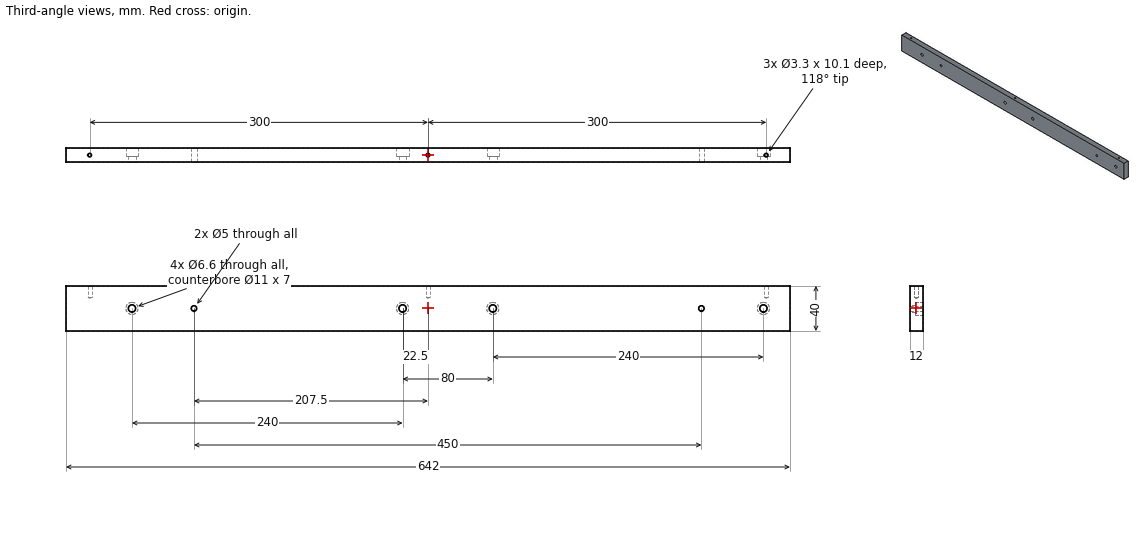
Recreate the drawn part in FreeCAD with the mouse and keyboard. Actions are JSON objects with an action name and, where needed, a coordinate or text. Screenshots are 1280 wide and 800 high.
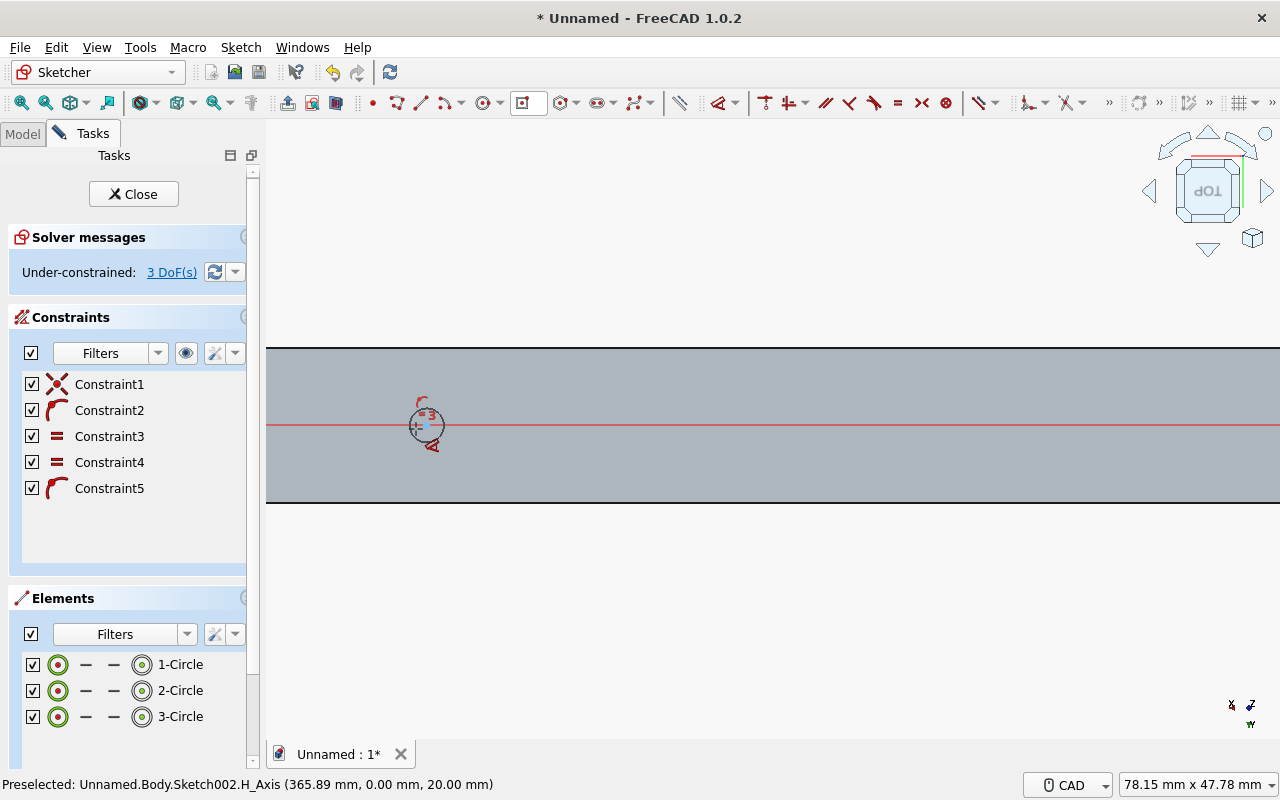
{"action": "left_click", "coordinate": [410, 425]}
{"action": "left_click", "coordinate": [385, 401]}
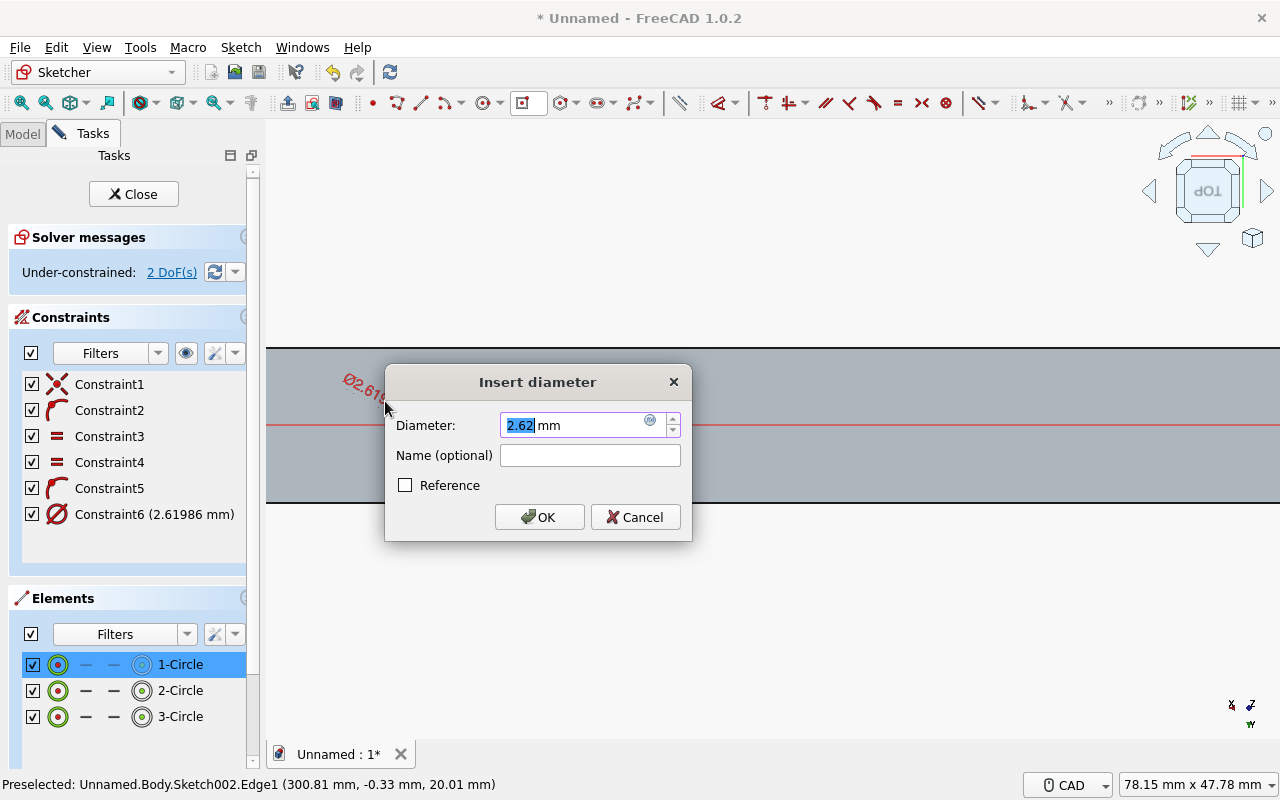
{"action": "type", "text": "3.3"}
{"action": "key", "text": "Return"}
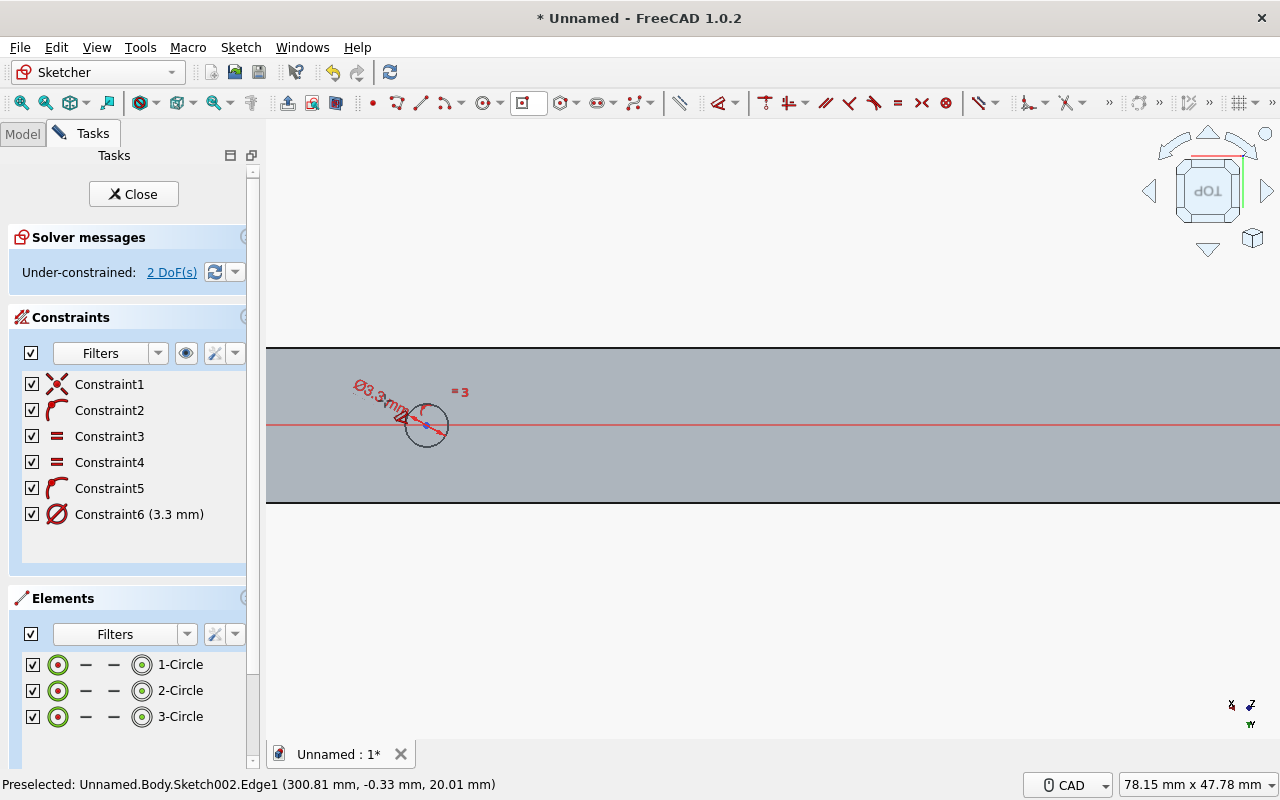
{"action": "scroll", "coordinate": [415, 429], "scroll_direction": "down", "scroll_amount": 13}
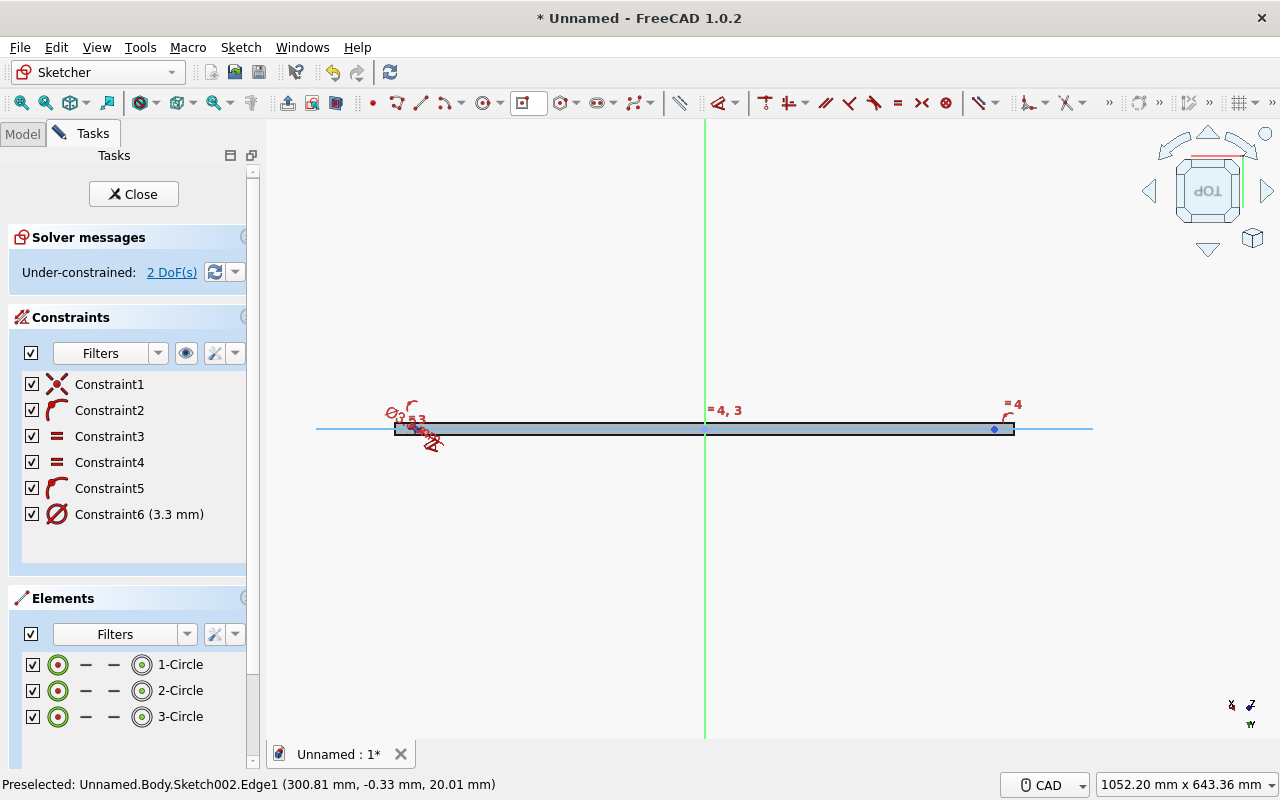
{"action": "left_click", "coordinate": [416, 429]}
{"action": "left_click", "coordinate": [560, 463]}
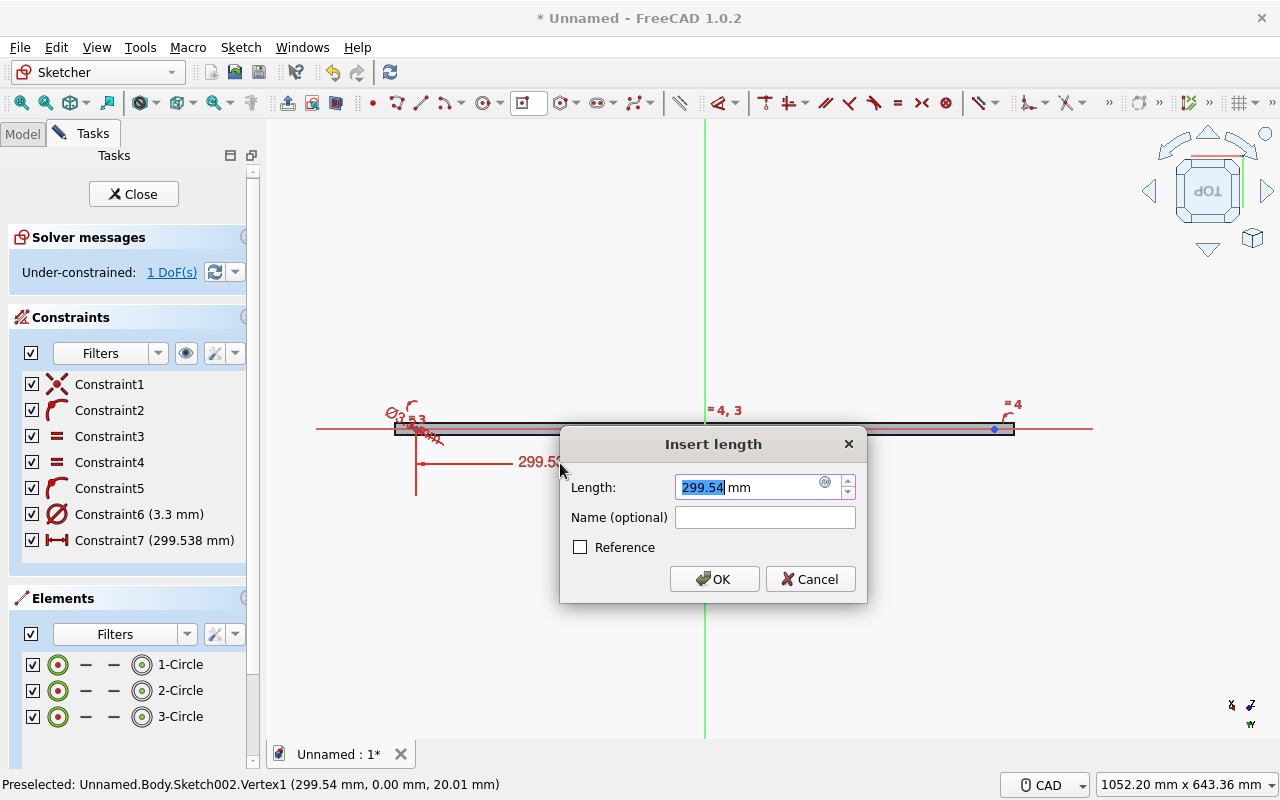
{"action": "type", "text": "300"}
{"action": "key", "text": "Return"}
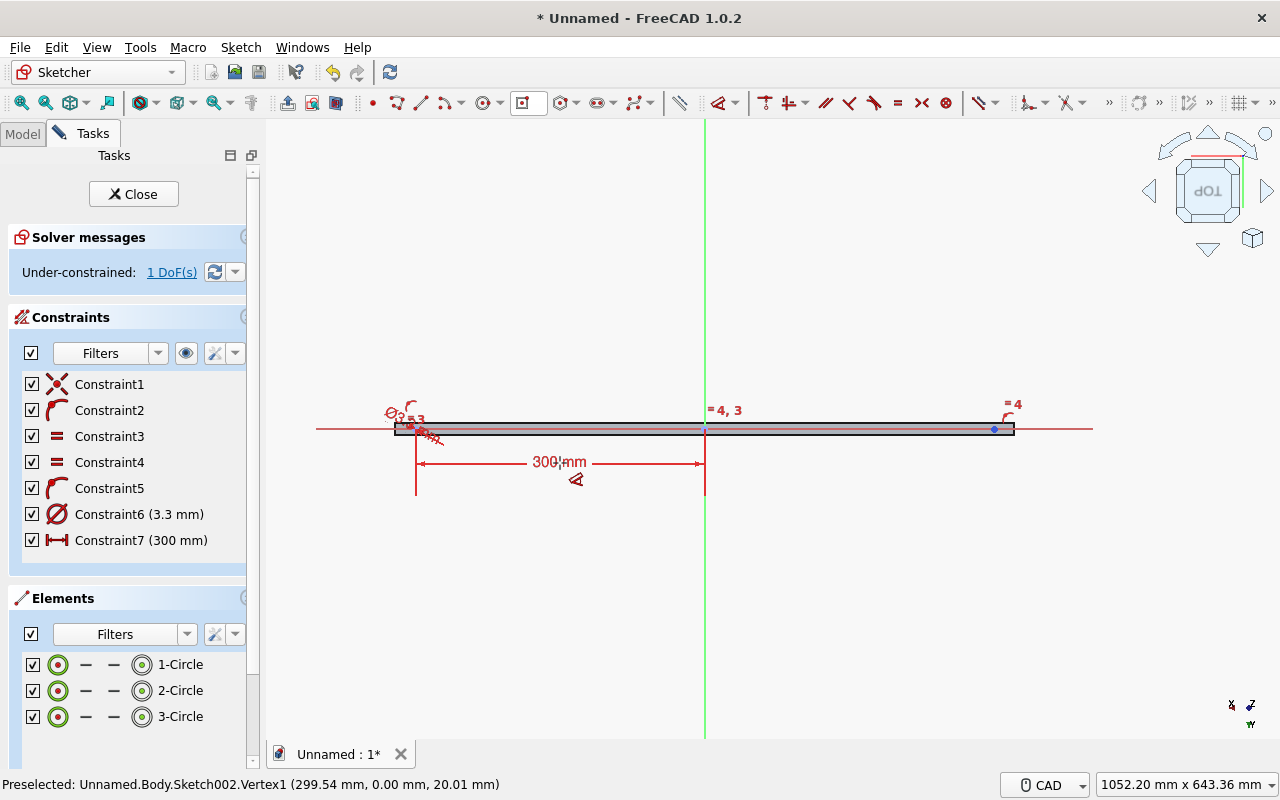
{"action": "left_click", "coordinate": [994, 429]}
{"action": "left_click", "coordinate": [849, 463]}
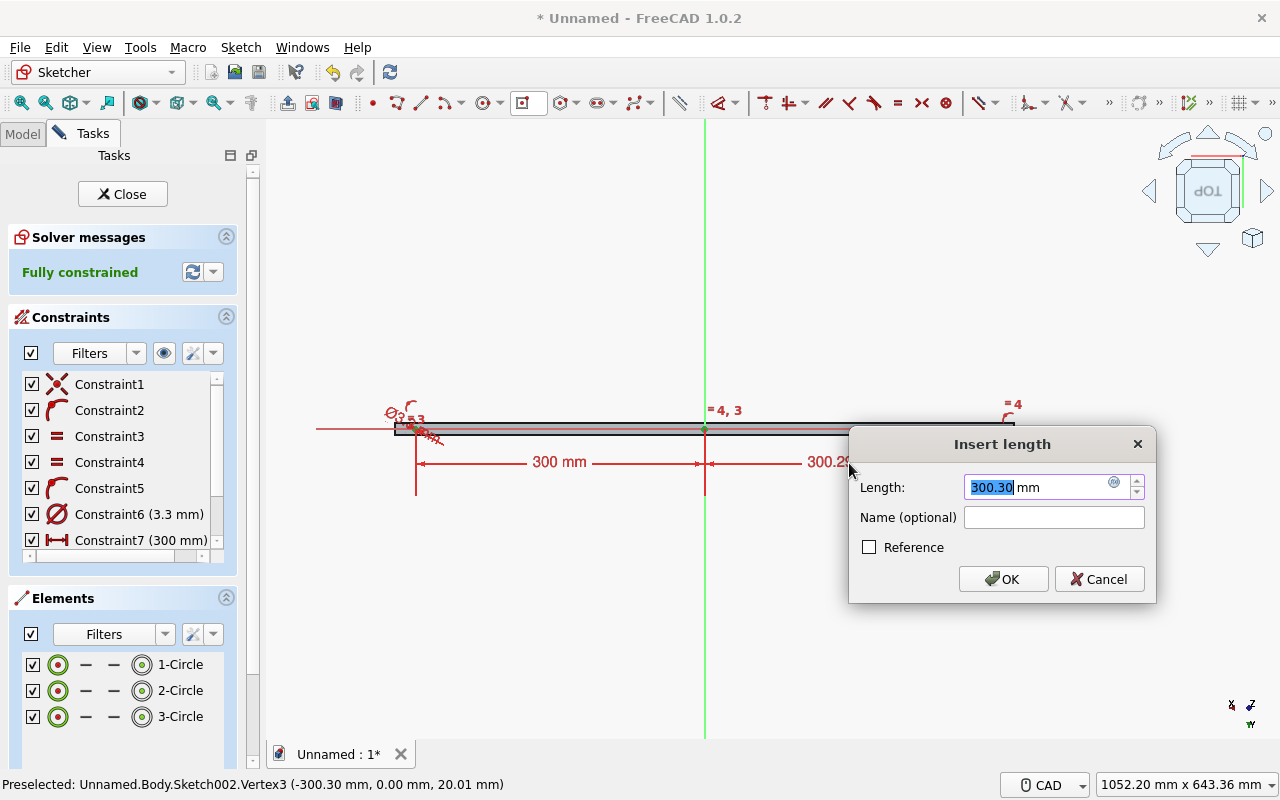
{"action": "type", "text": "300"}
{"action": "key", "text": "Return"}
{"action": "key", "text": "Escape"}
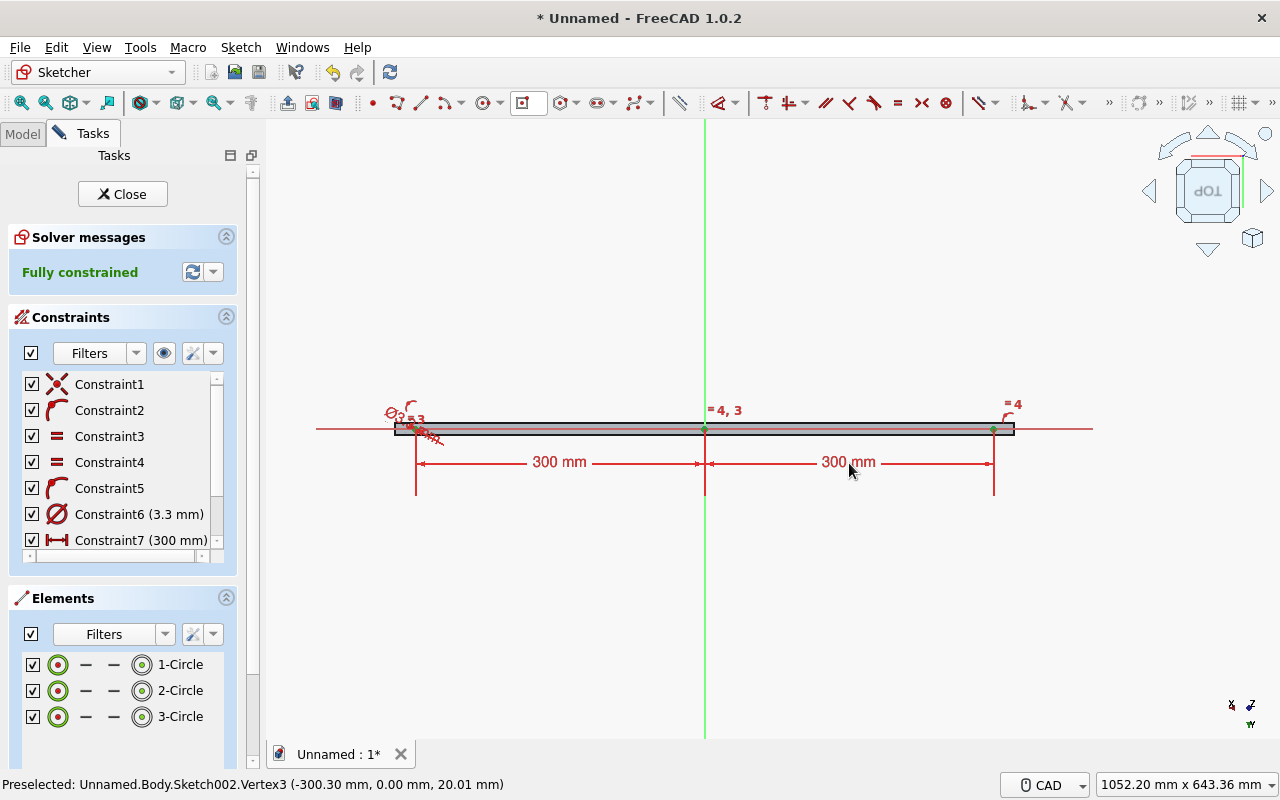
{"action": "left_click", "coordinate": [123, 194]}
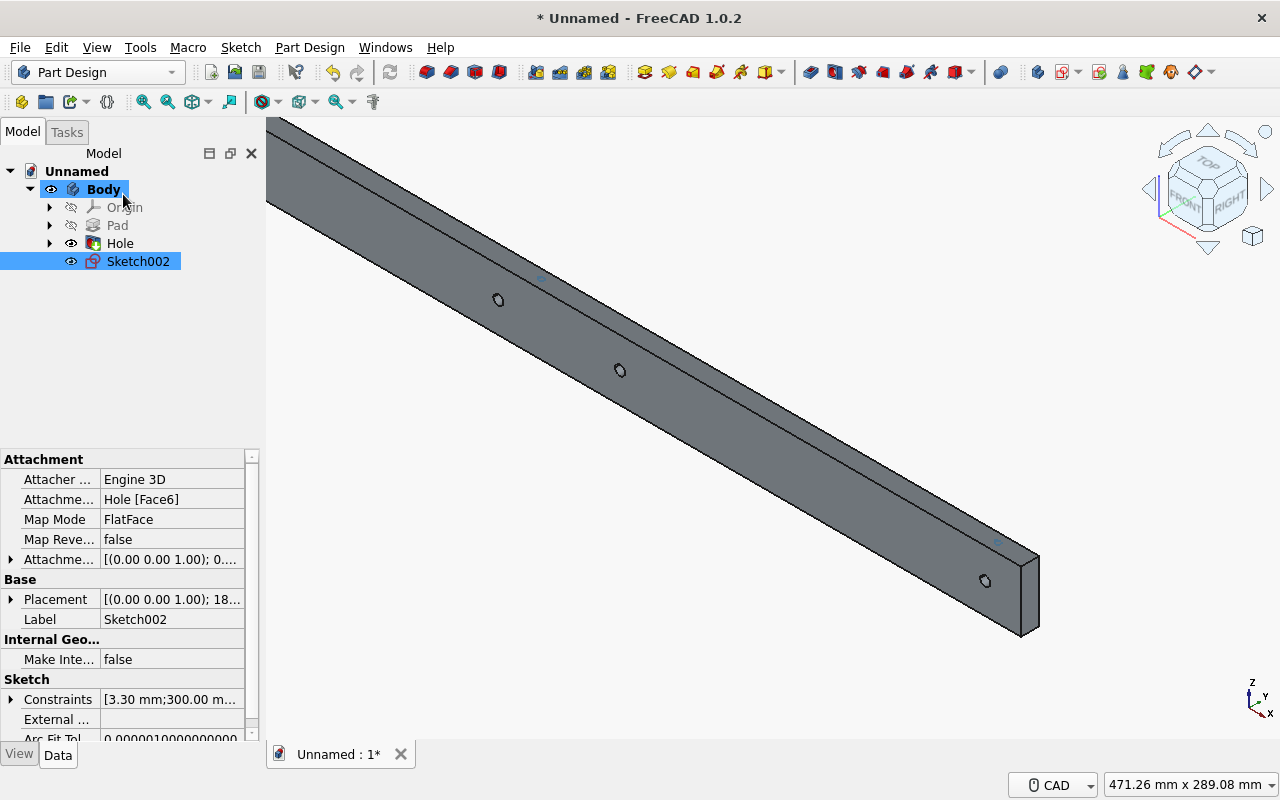
{"action": "left_click", "coordinate": [836, 72]}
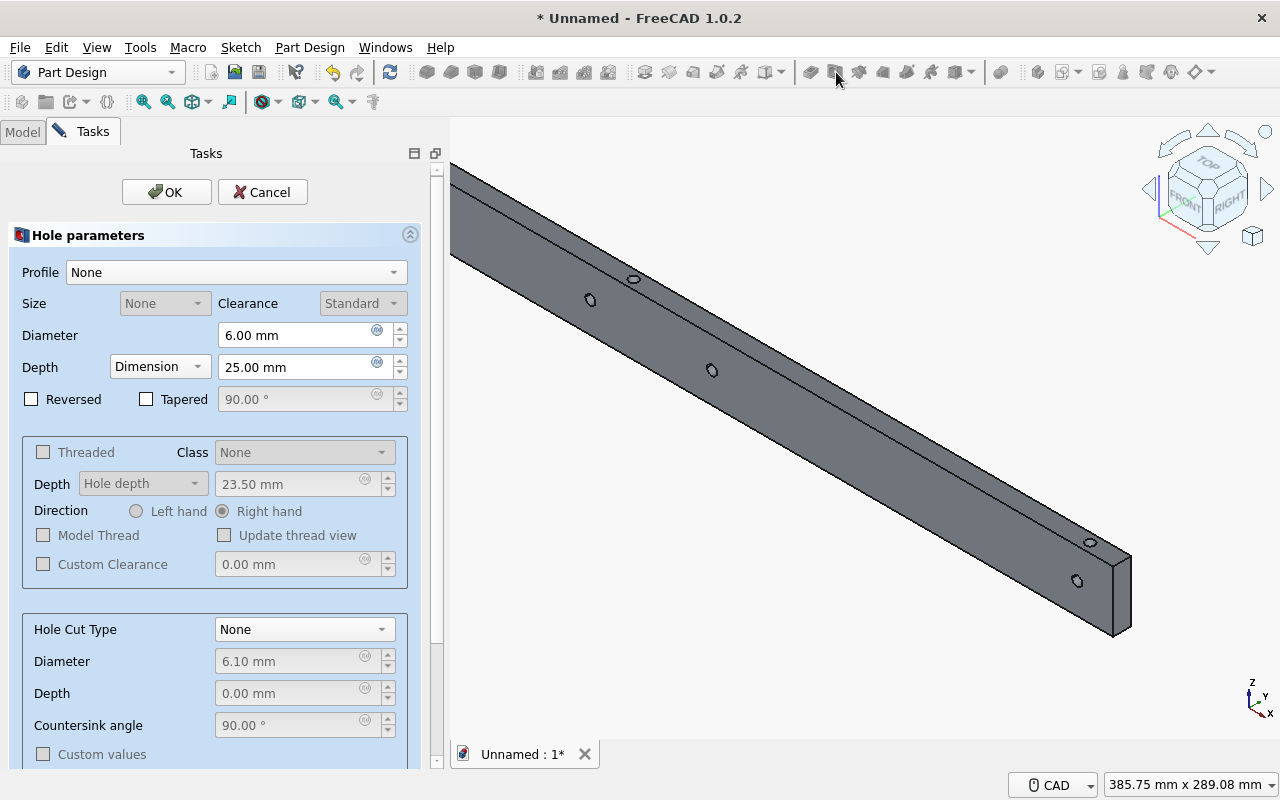
{"action": "triple_click", "coordinate": [305, 335]}